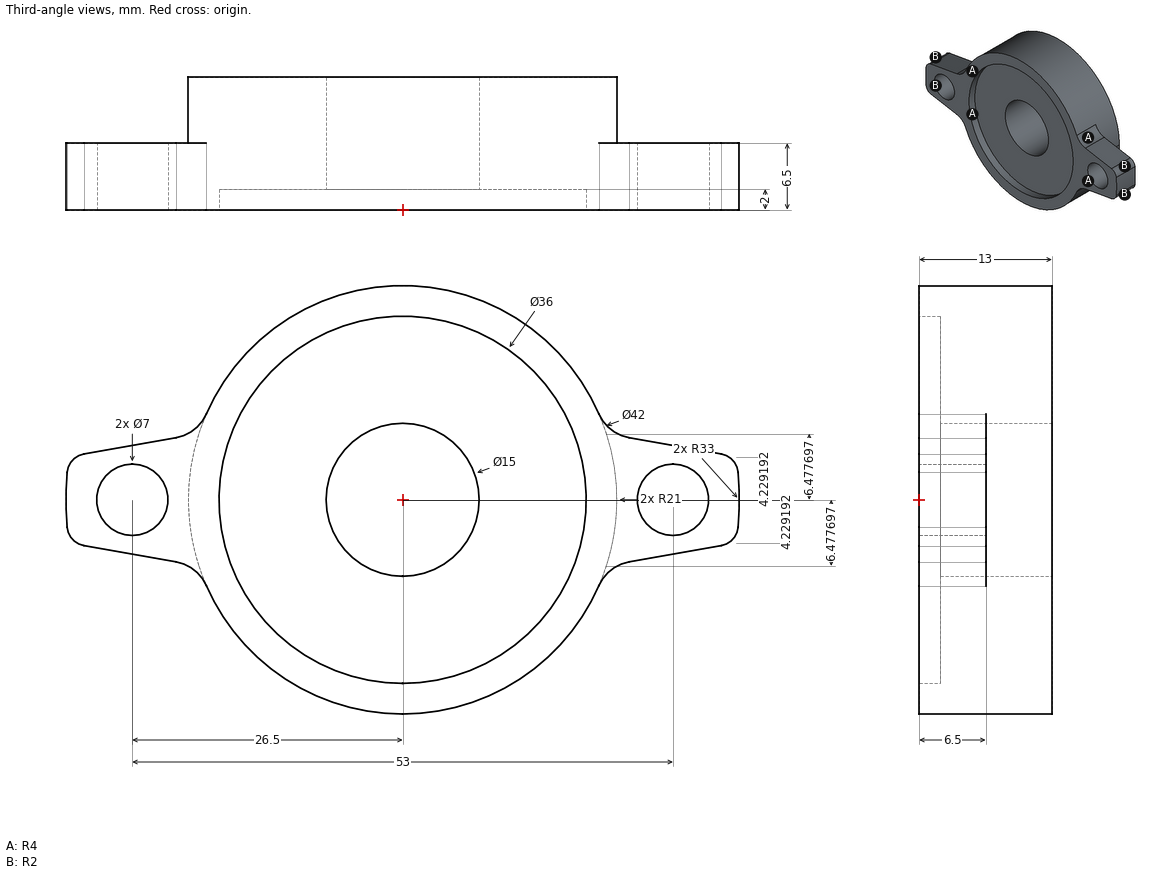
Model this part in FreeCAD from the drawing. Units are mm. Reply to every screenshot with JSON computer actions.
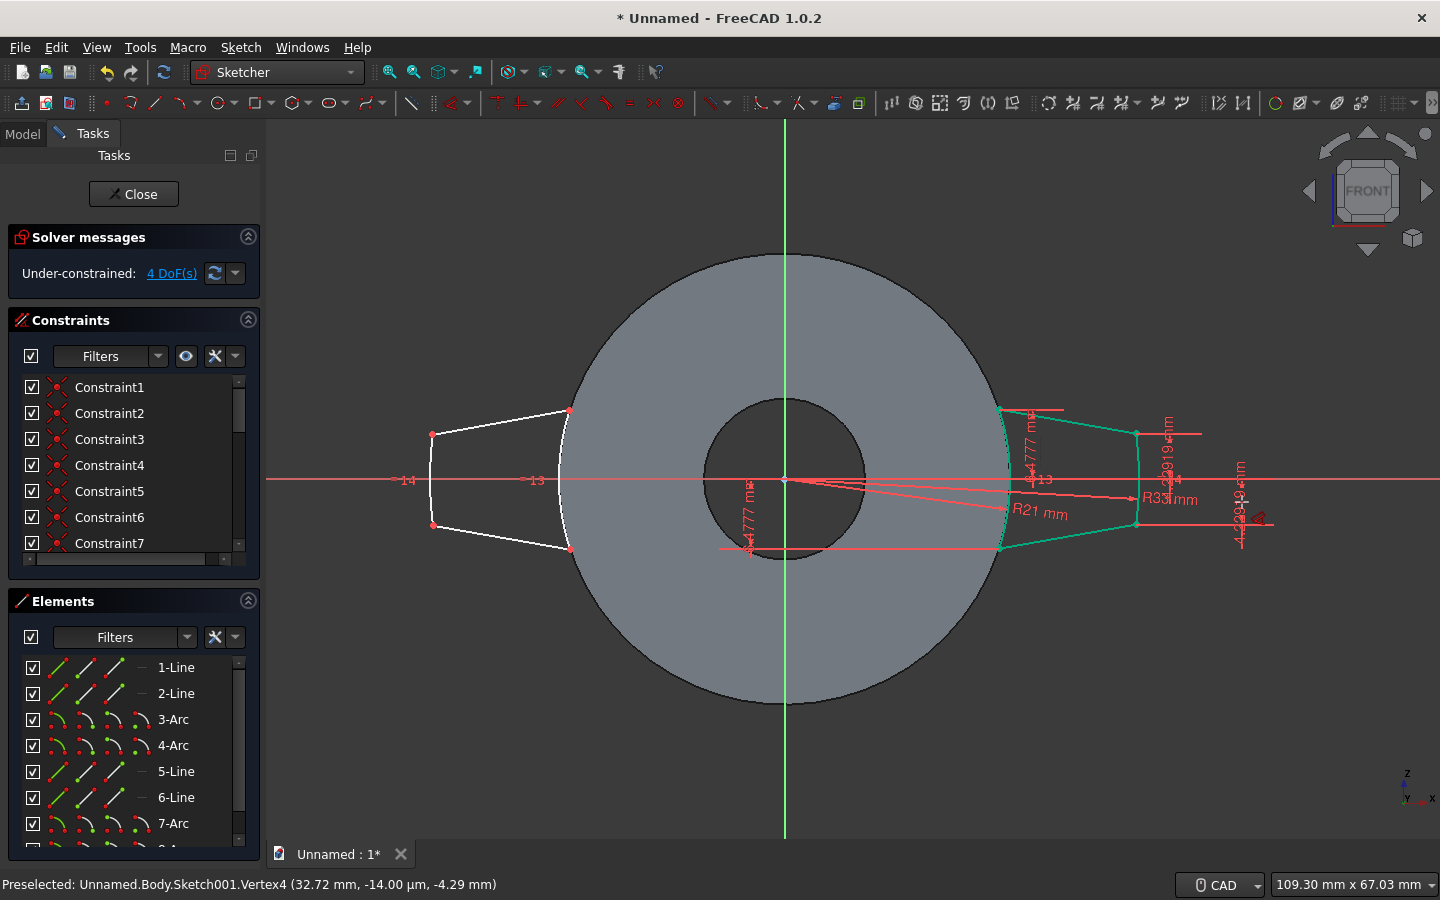
{"action": "left_click", "coordinate": [433, 526]}
{"action": "left_click", "coordinate": [399, 502]}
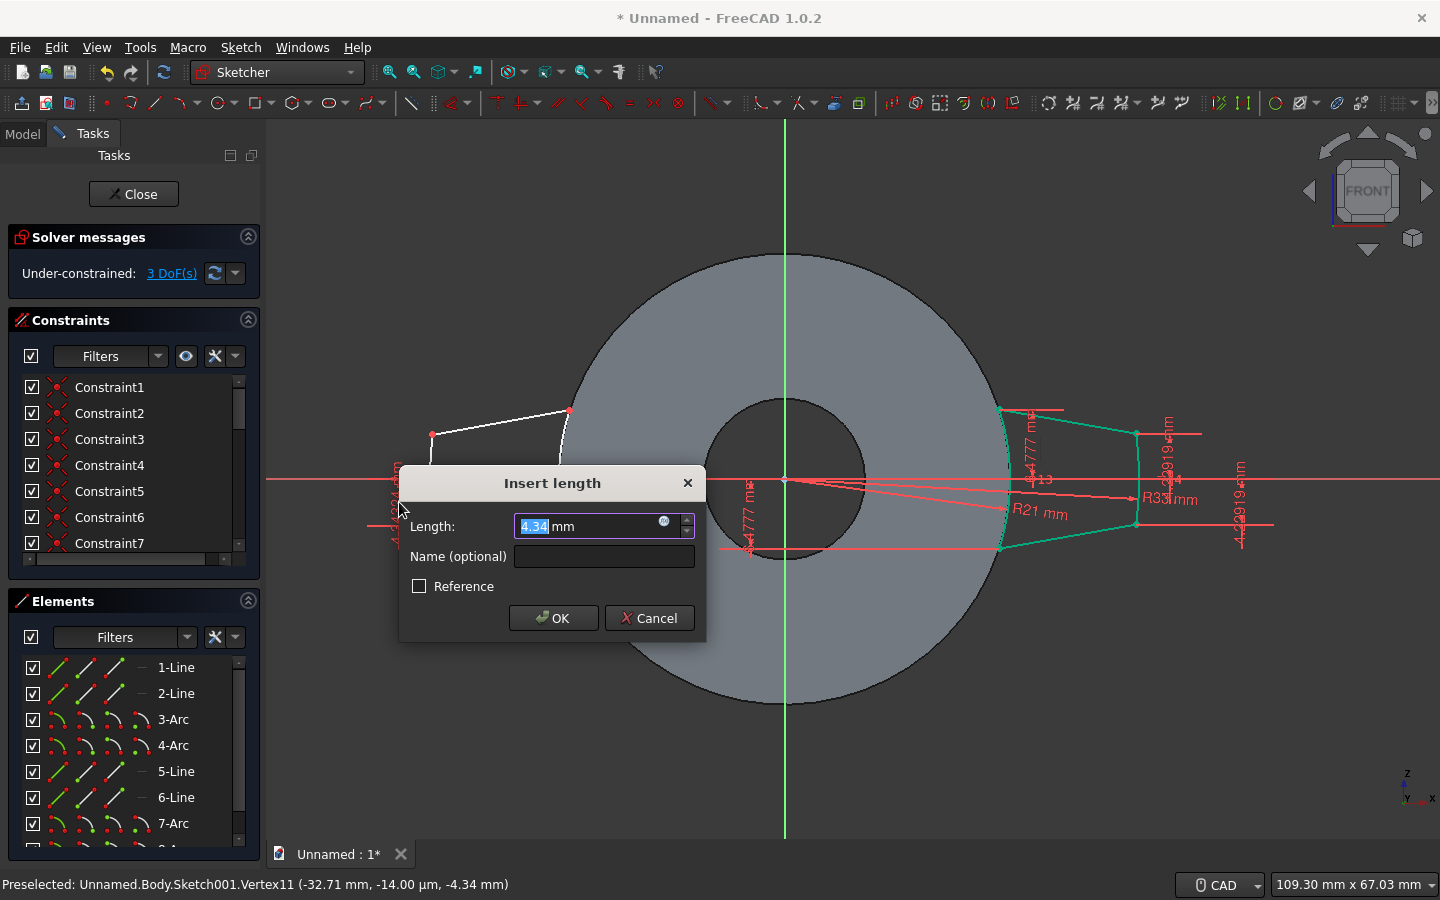
{"action": "type", "text": "4.229192"}
{"action": "key", "text": "Return"}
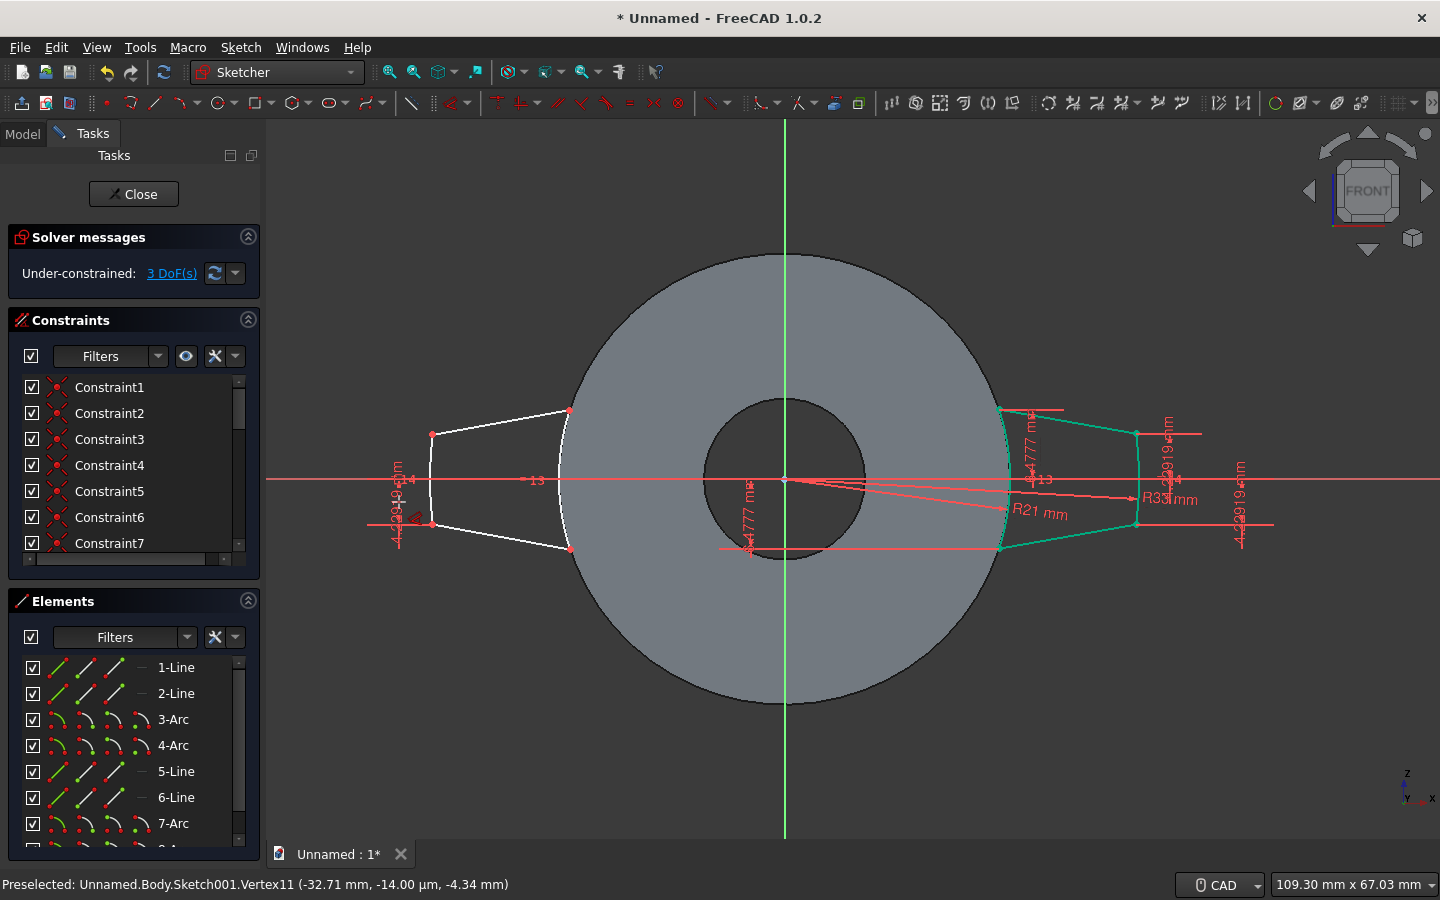
{"action": "left_click", "coordinate": [570, 550]}
{"action": "left_click", "coordinate": [536, 514]}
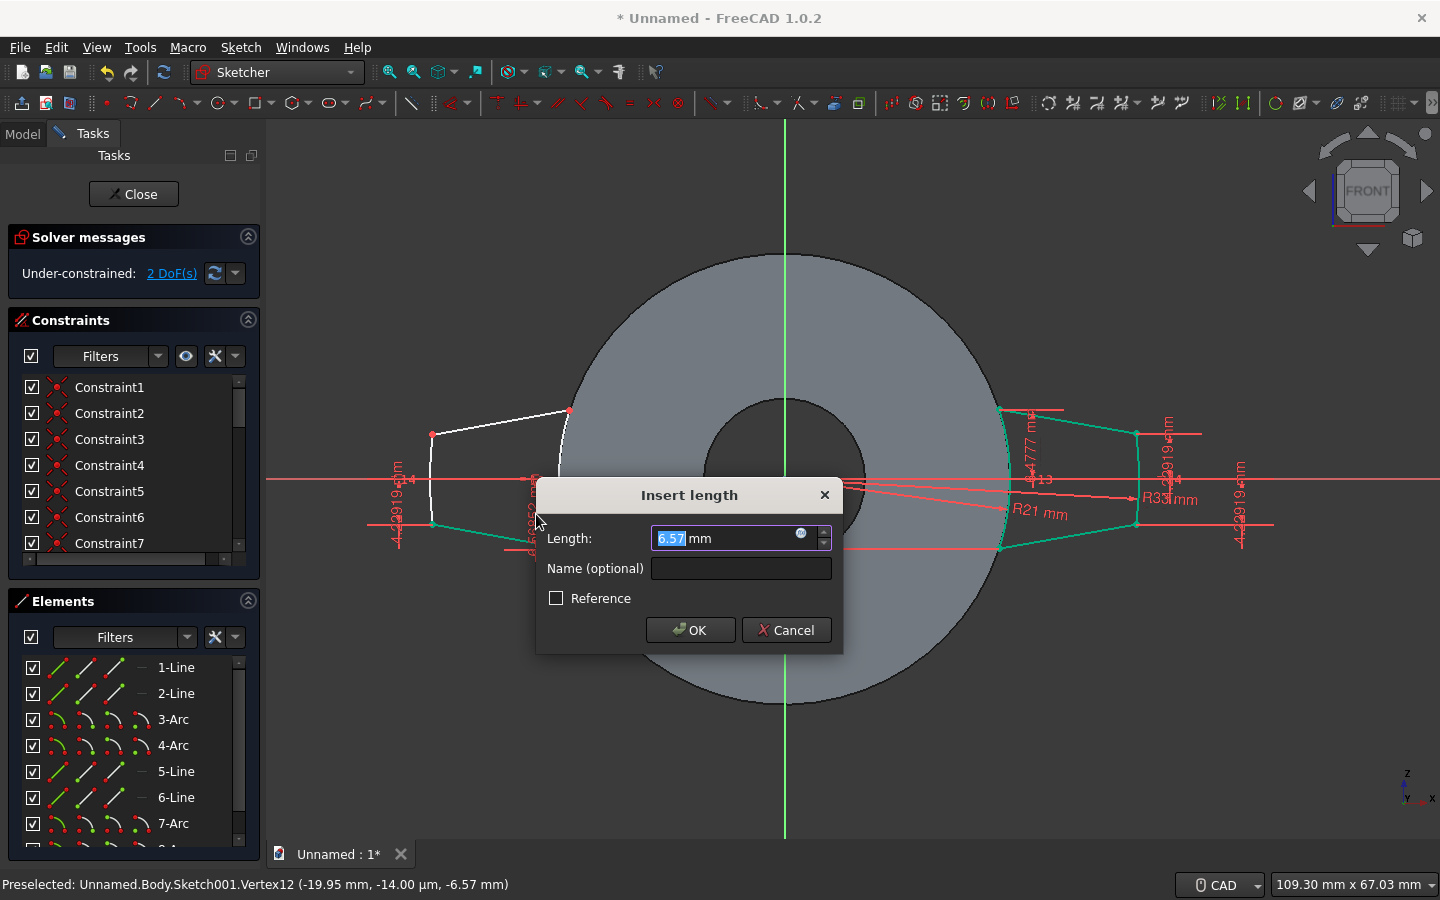
{"action": "type", "text": "6.477697"}
{"action": "key", "text": "Return"}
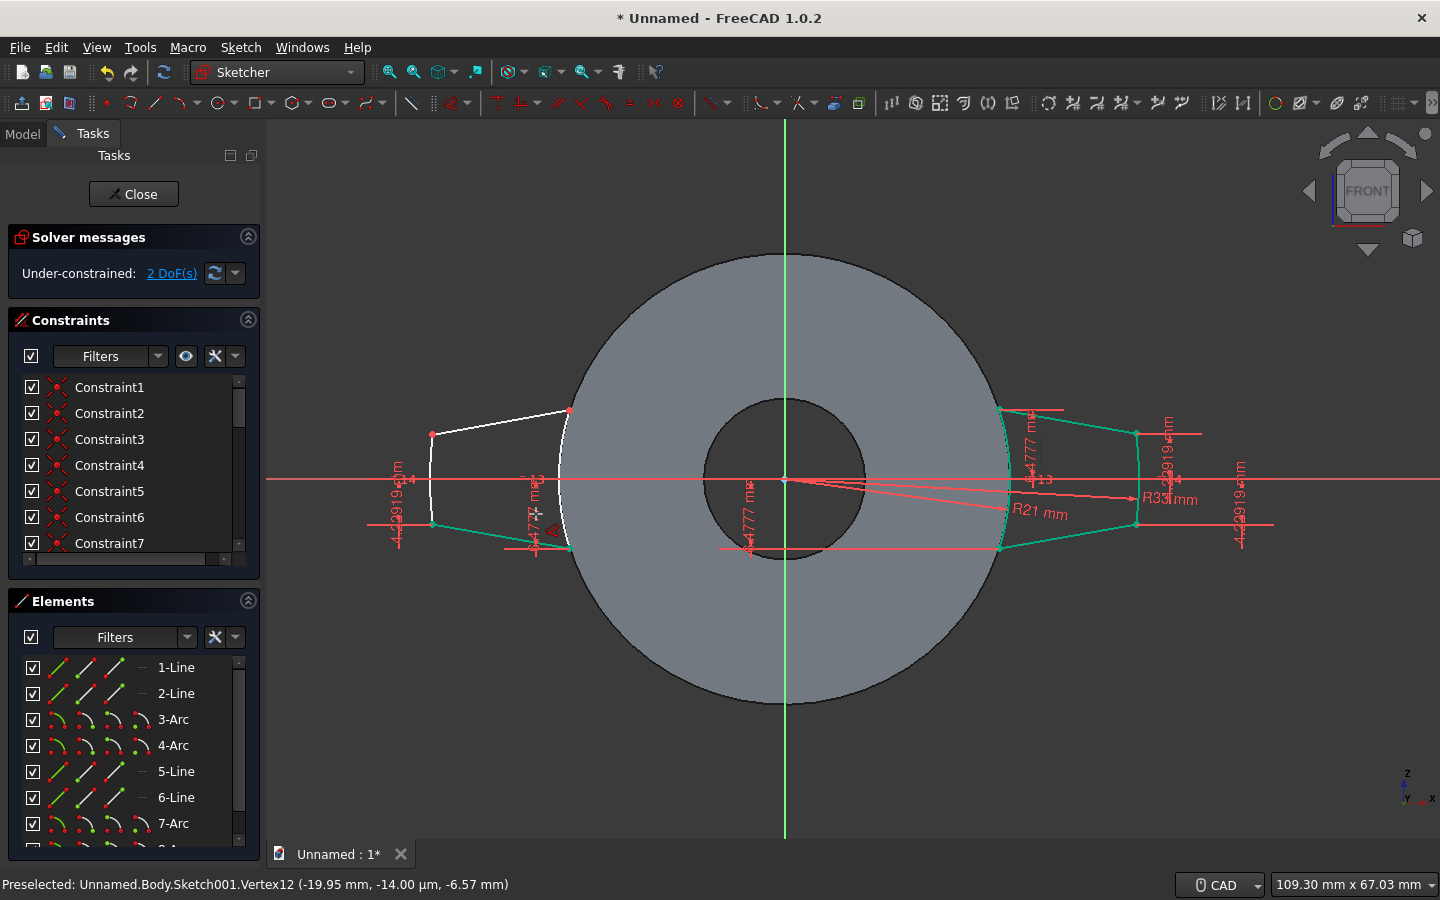
{"action": "left_click", "coordinate": [570, 410]}
{"action": "left_click", "coordinate": [536, 445]}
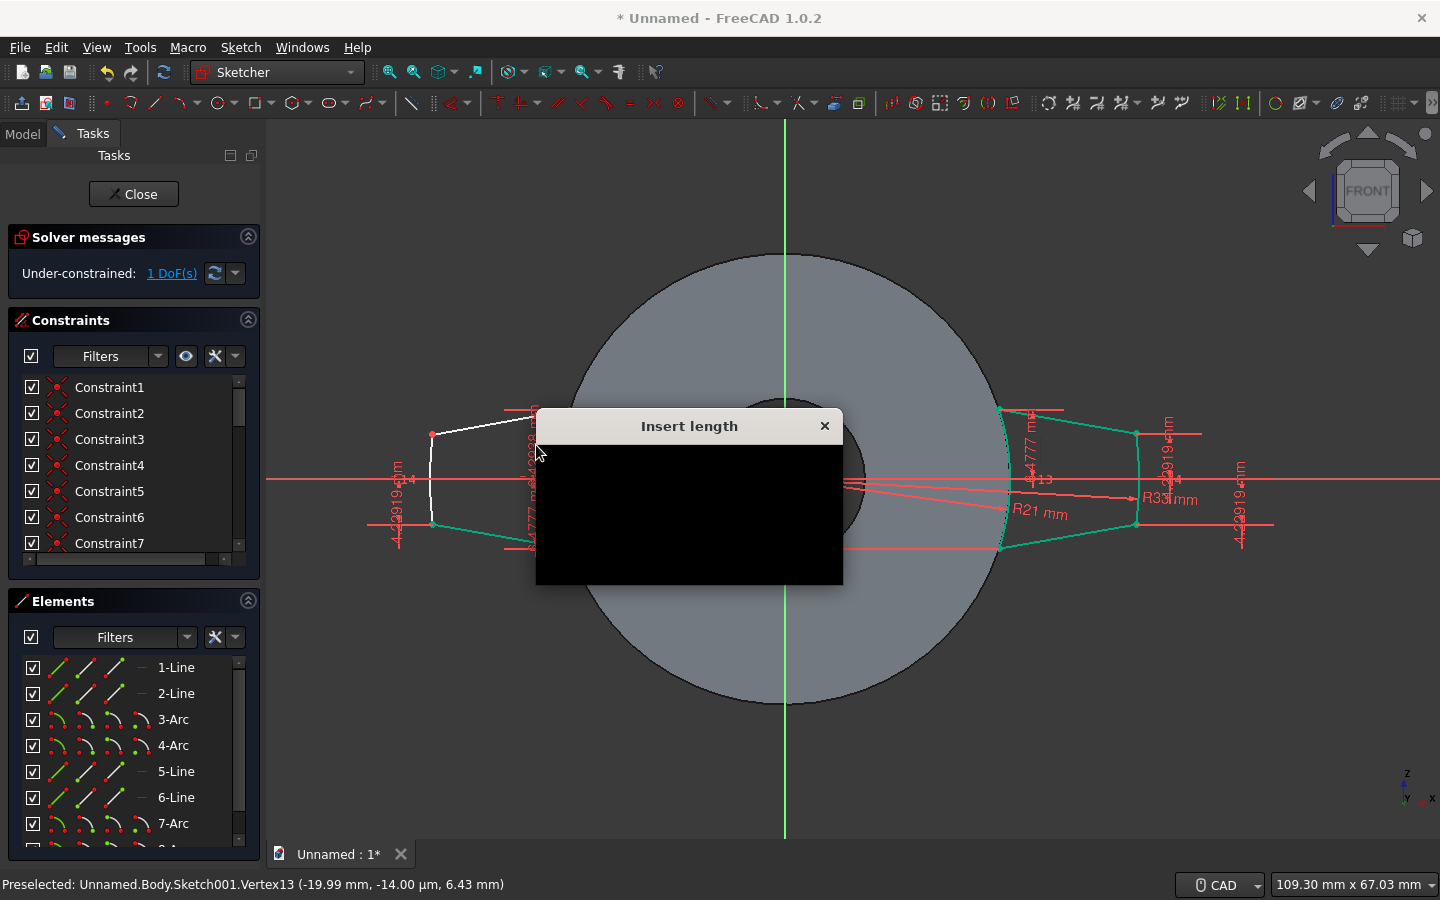
{"action": "type", "text": "6.477697"}
{"action": "key", "text": "Return"}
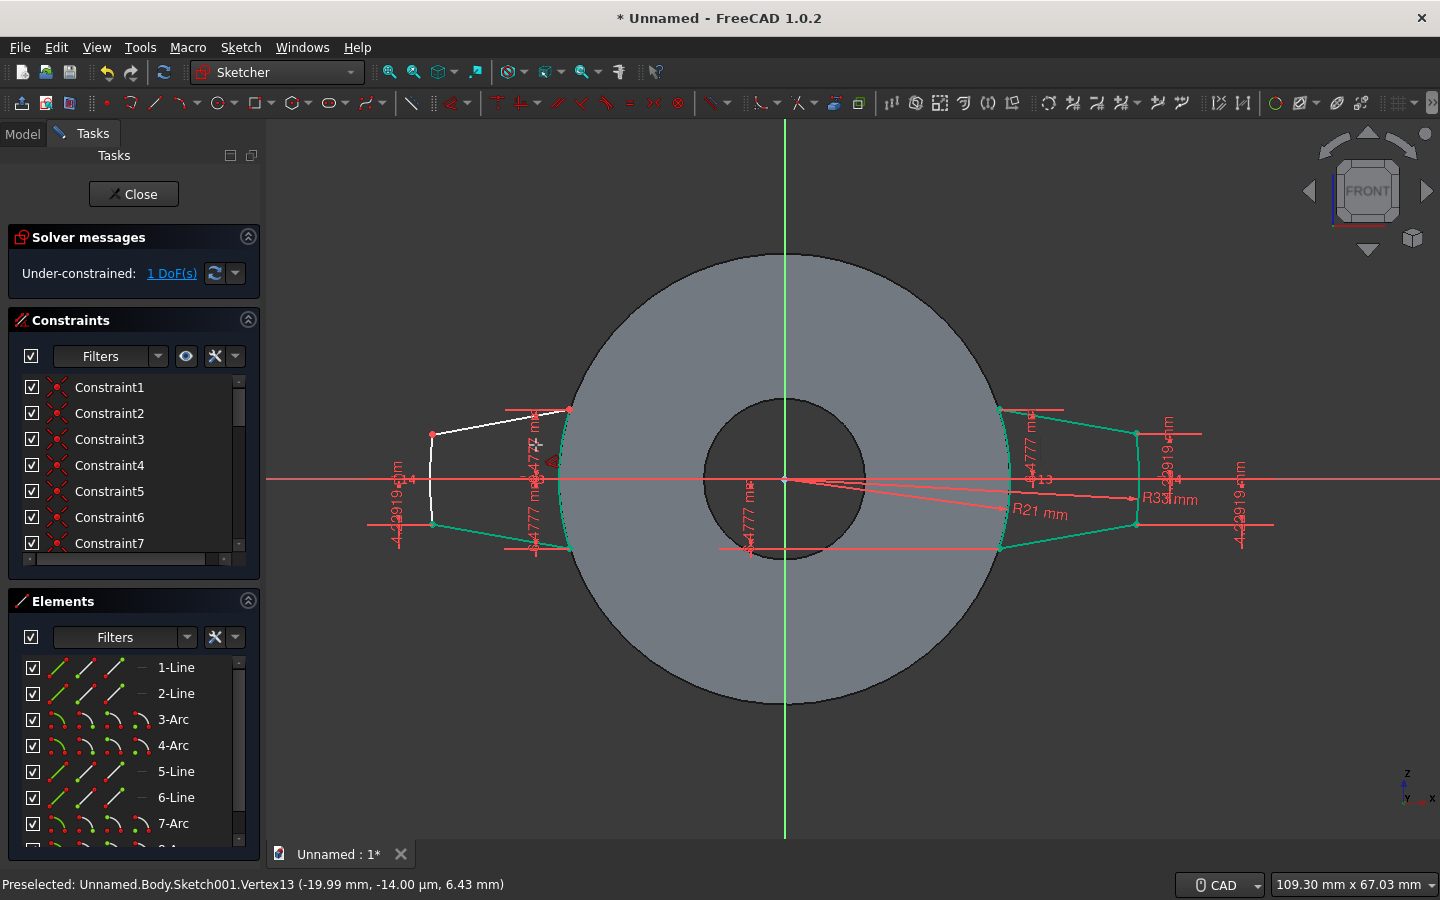
{"action": "left_click", "coordinate": [433, 435]}
{"action": "left_click", "coordinate": [399, 457]}